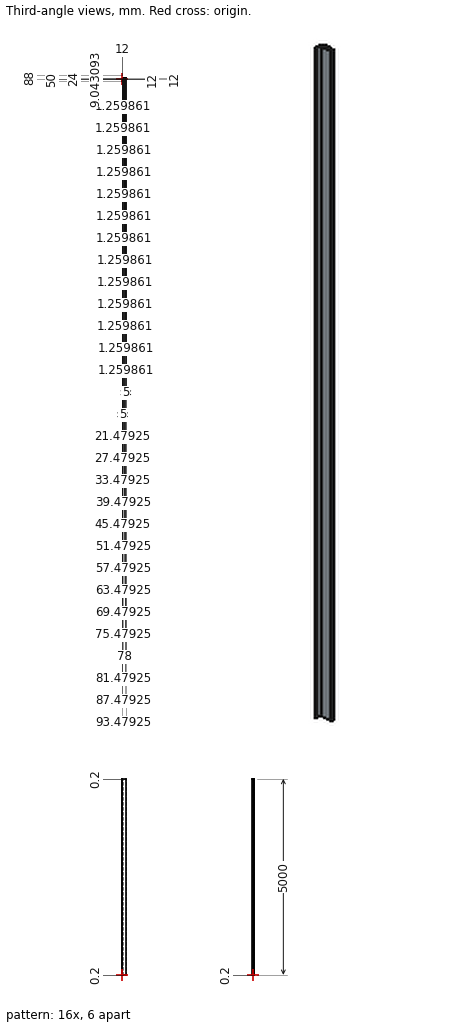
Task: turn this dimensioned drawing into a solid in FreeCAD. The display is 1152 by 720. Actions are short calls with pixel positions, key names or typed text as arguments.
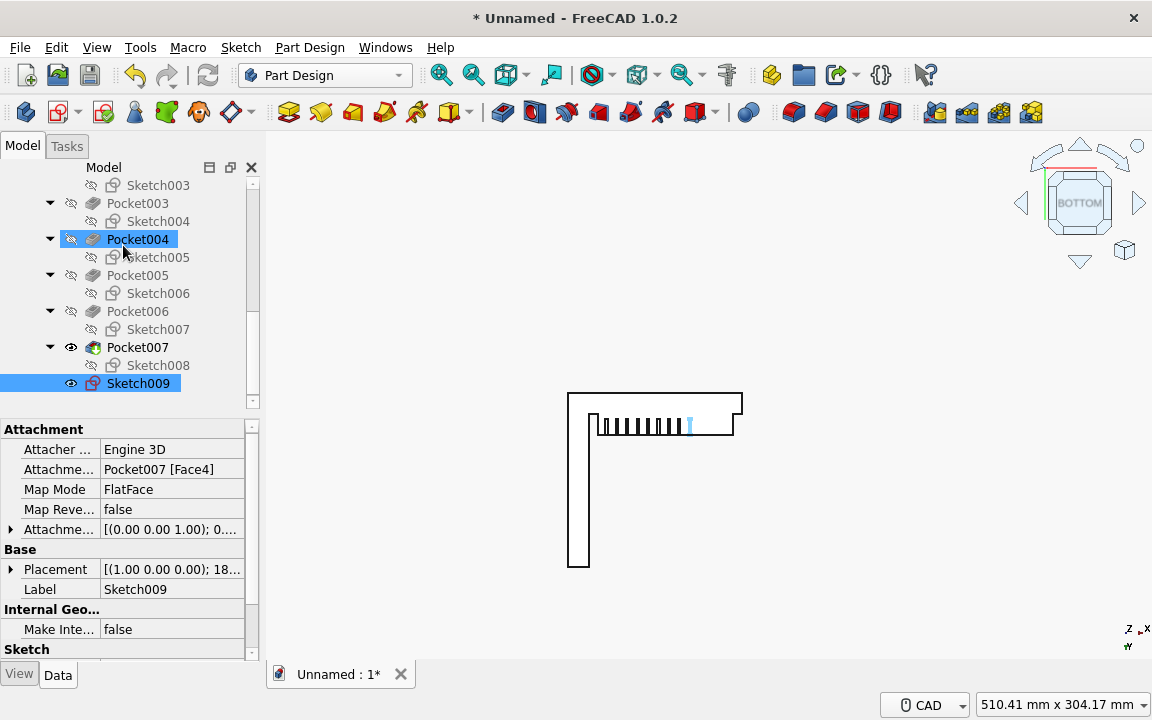
click(504, 112)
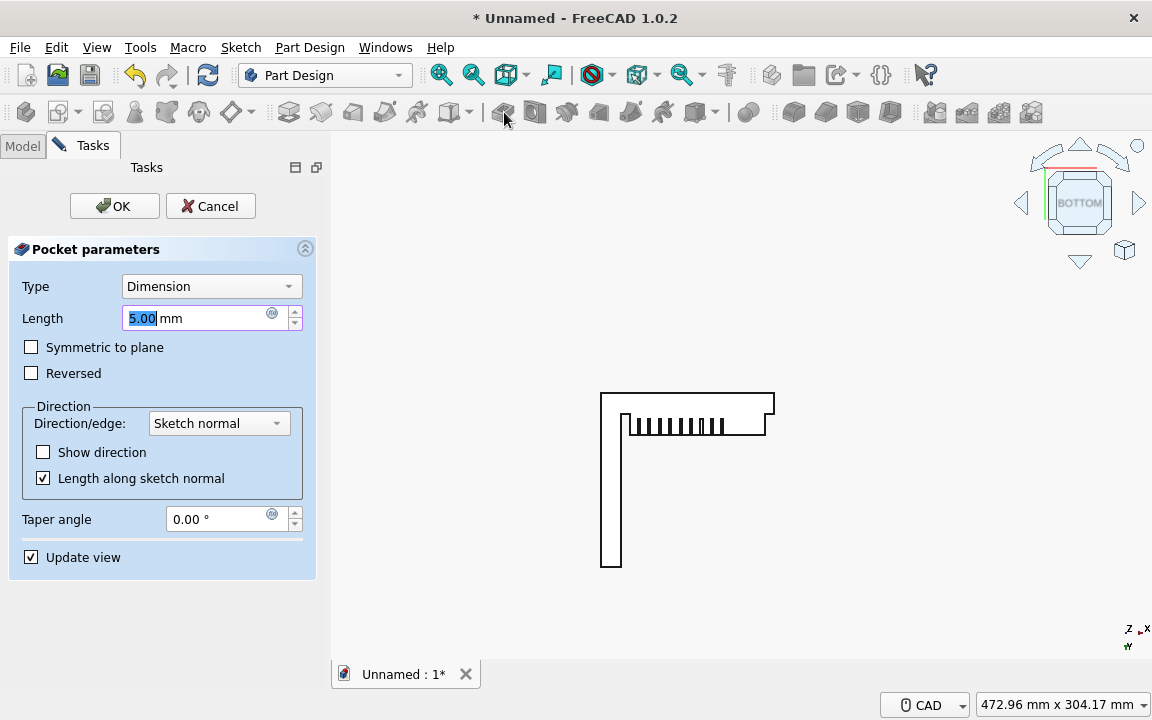
text(0.2)
key(Tab)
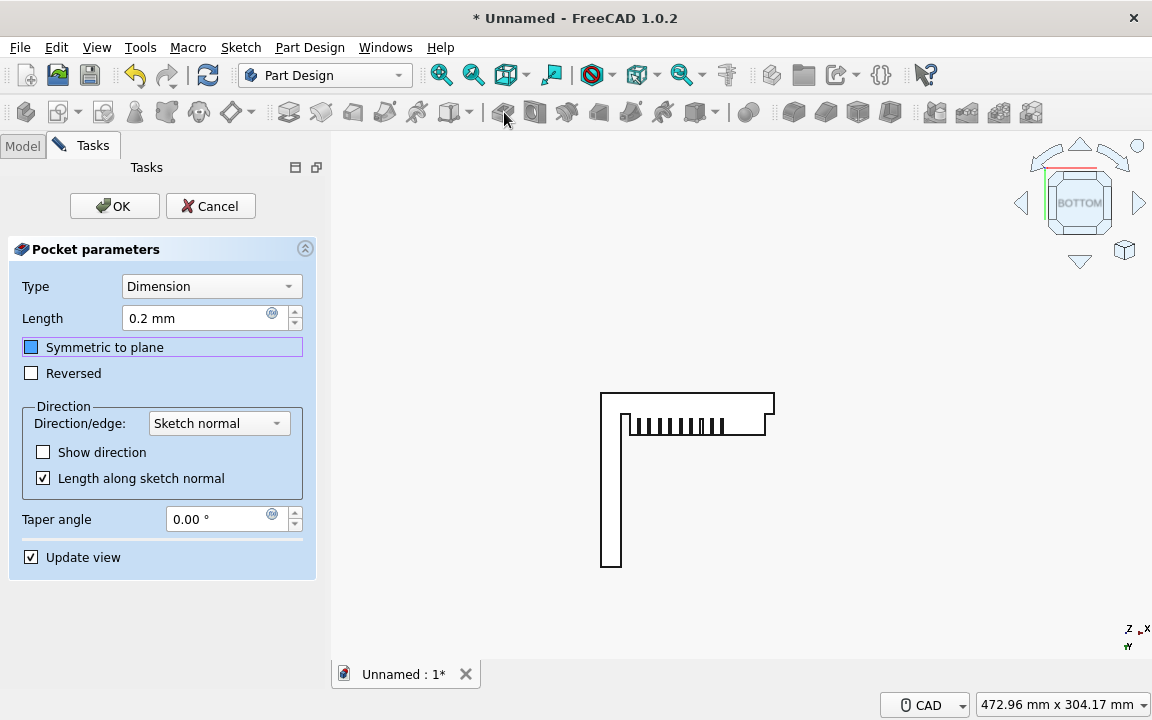
click(115, 206)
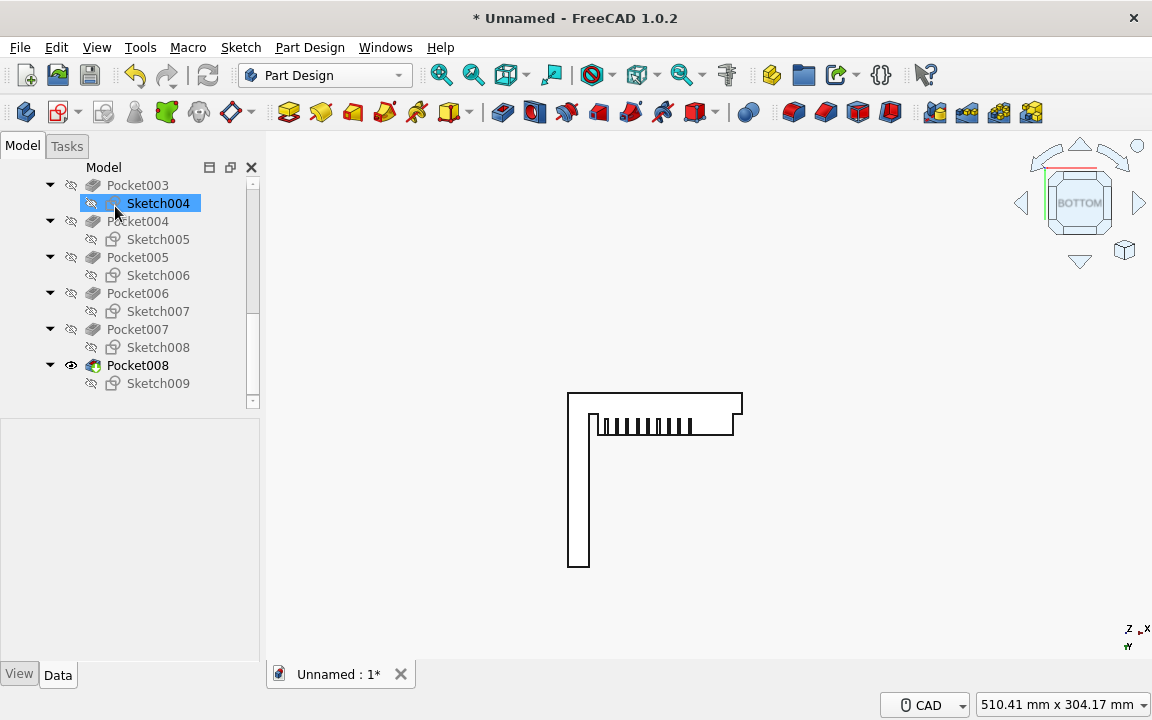
click(442, 76)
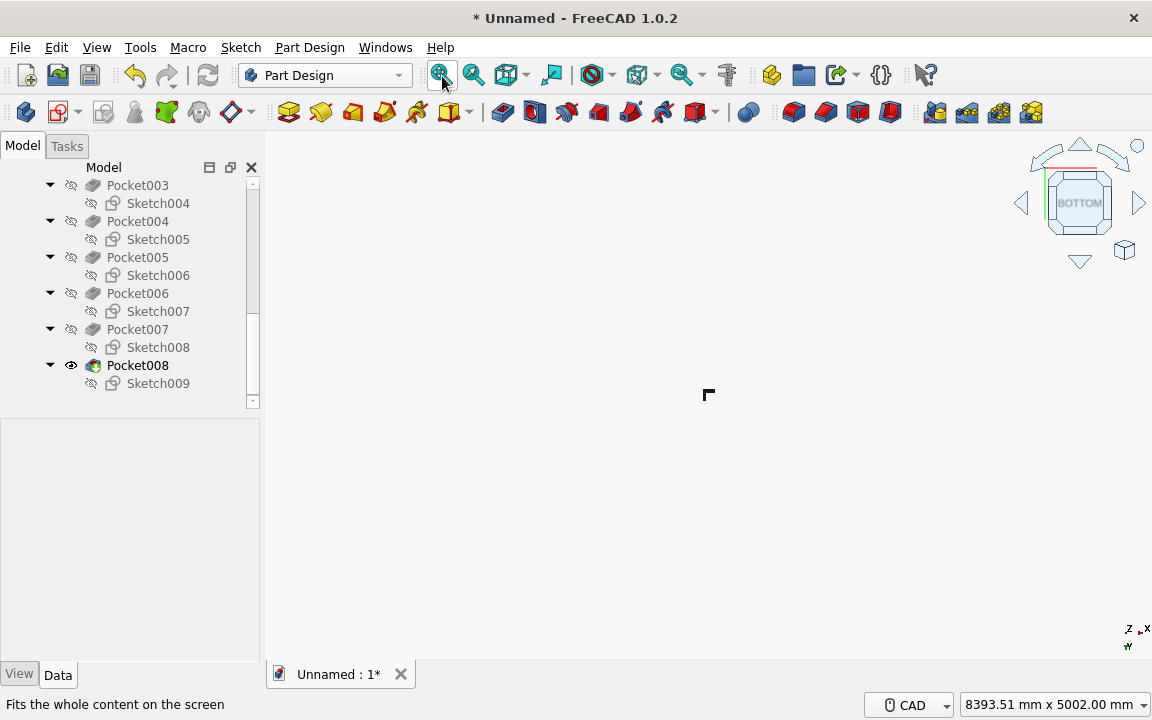
click(58, 112)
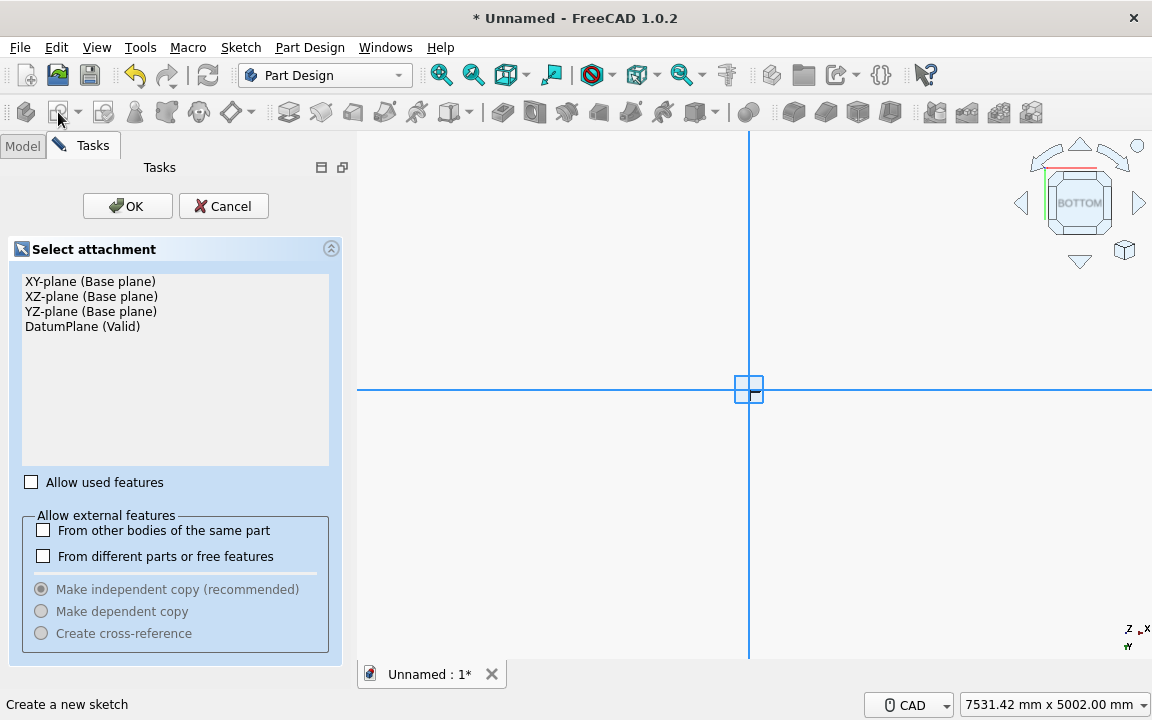
click(82, 282)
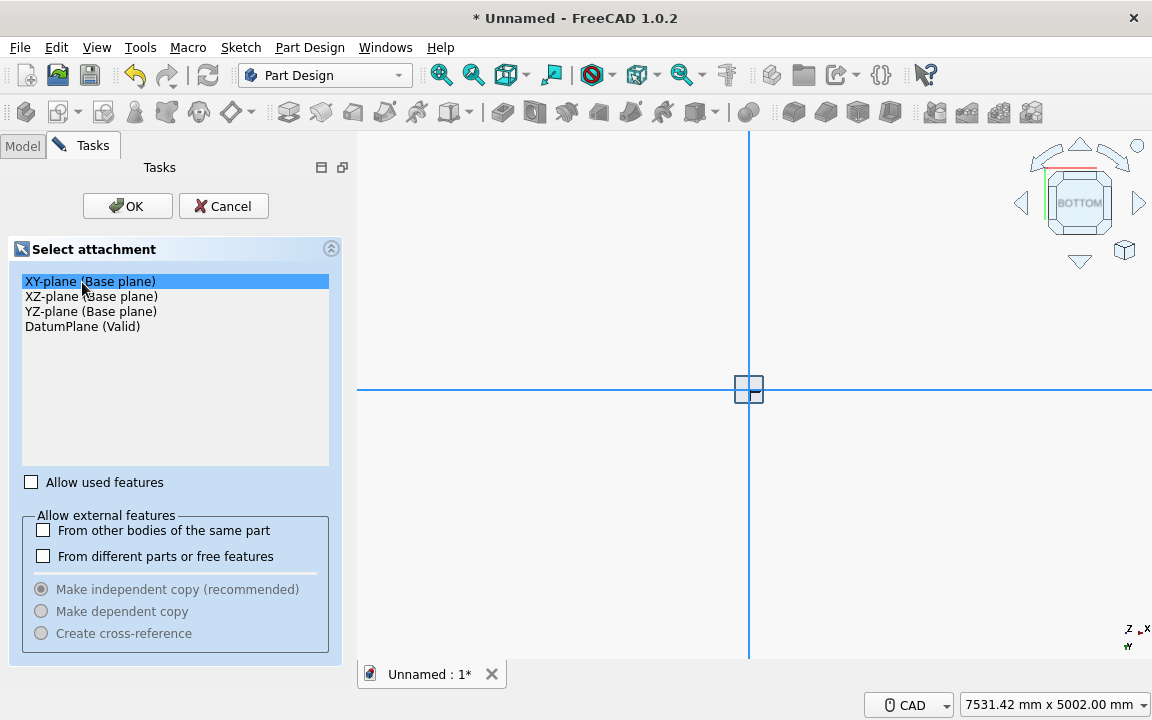
click(128, 206)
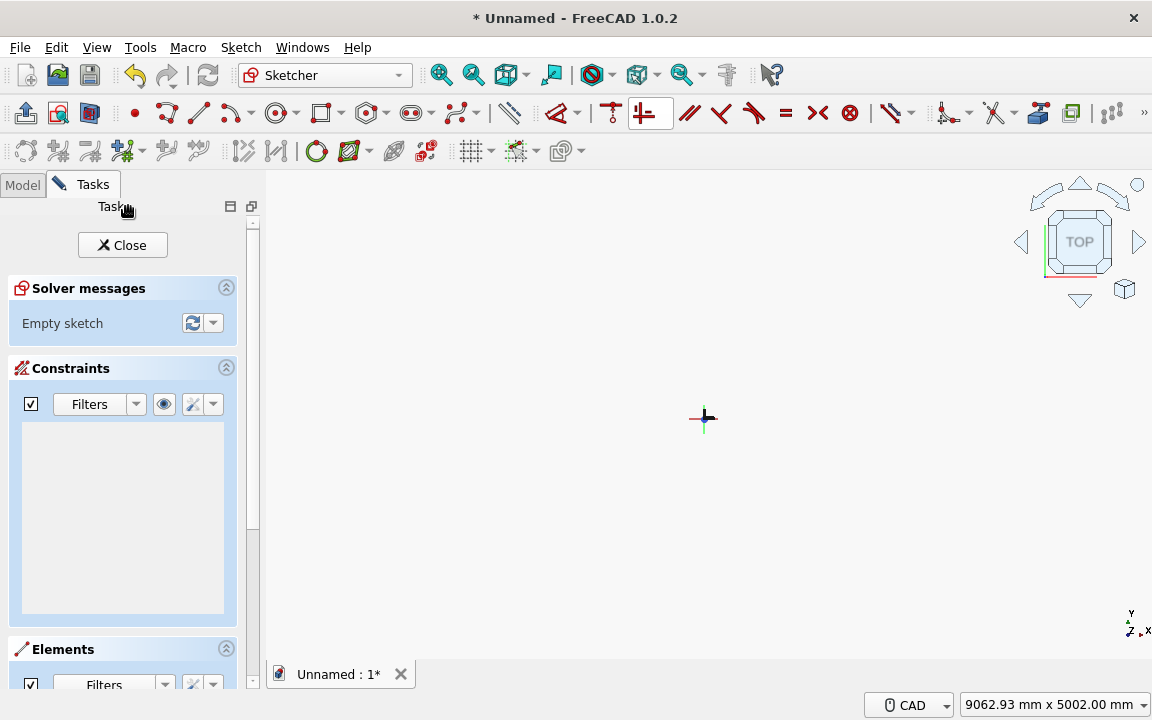
click(90, 114)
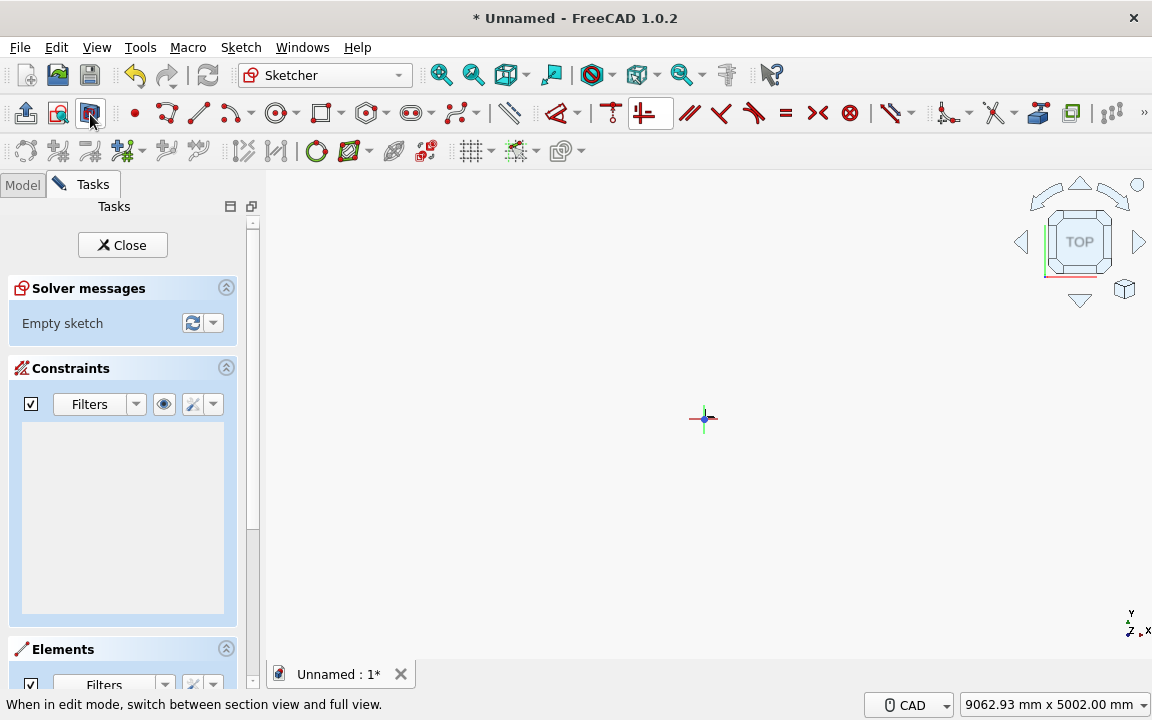
scroll(715, 418, up, 15)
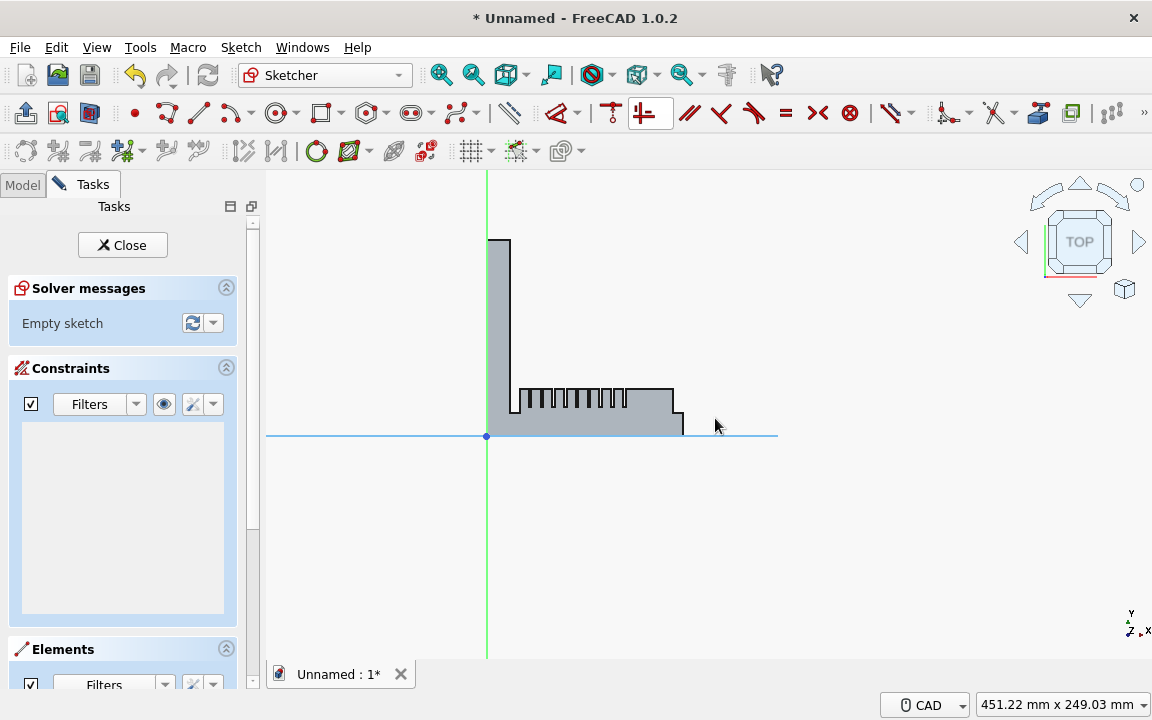
scroll(636, 397, up, 14)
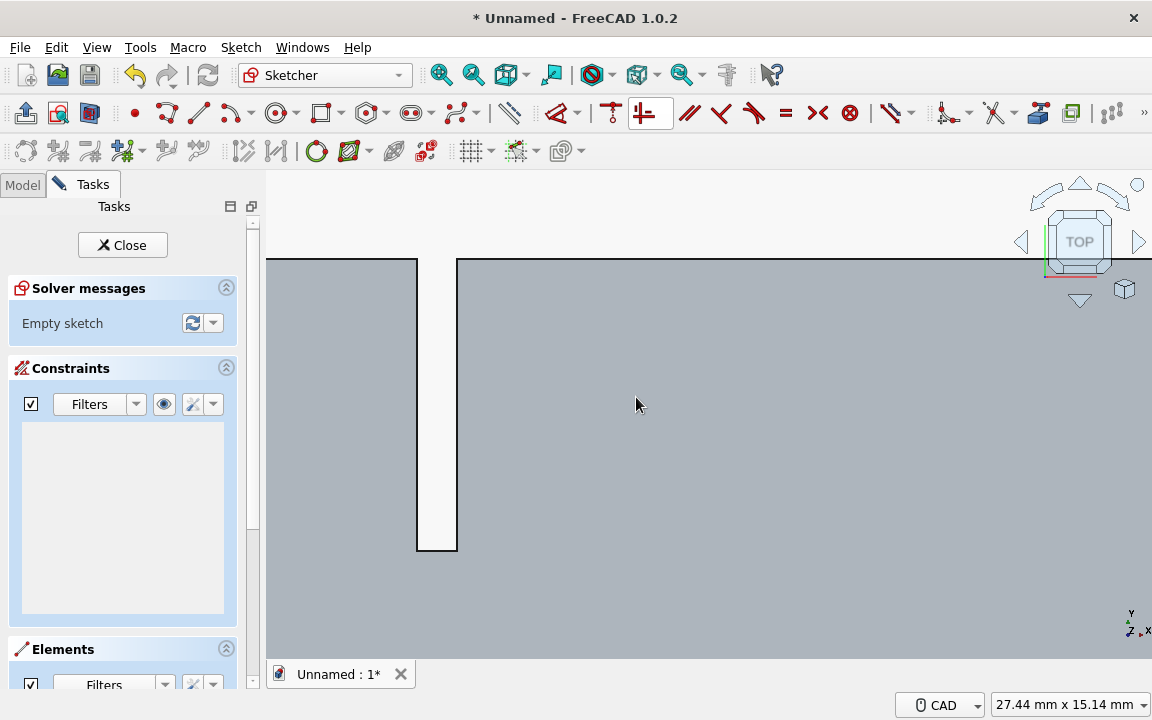
click(322, 114)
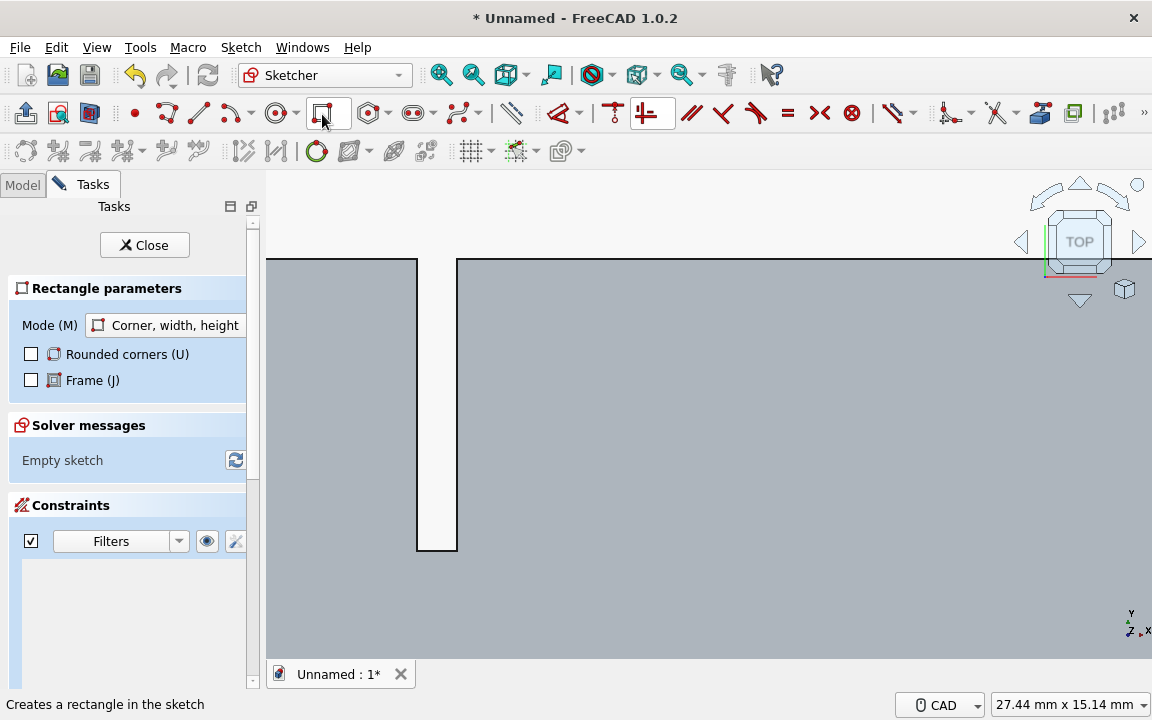
click(610, 259)
click(651, 551)
key(Escape)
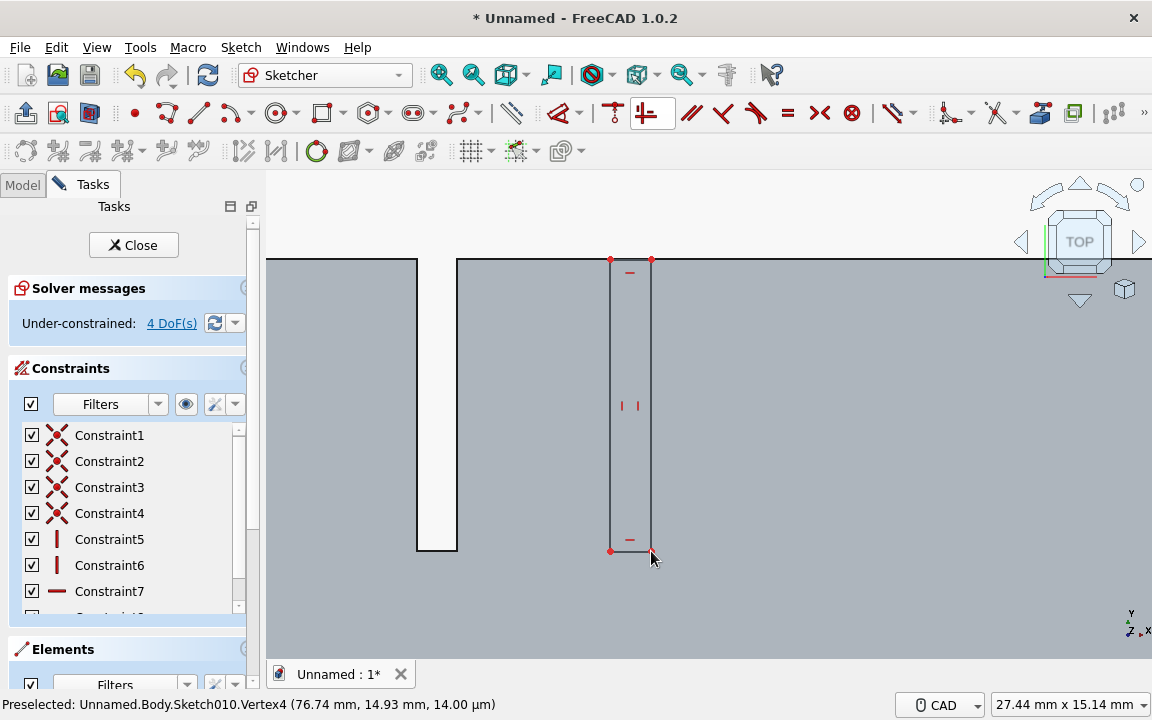
click(558, 114)